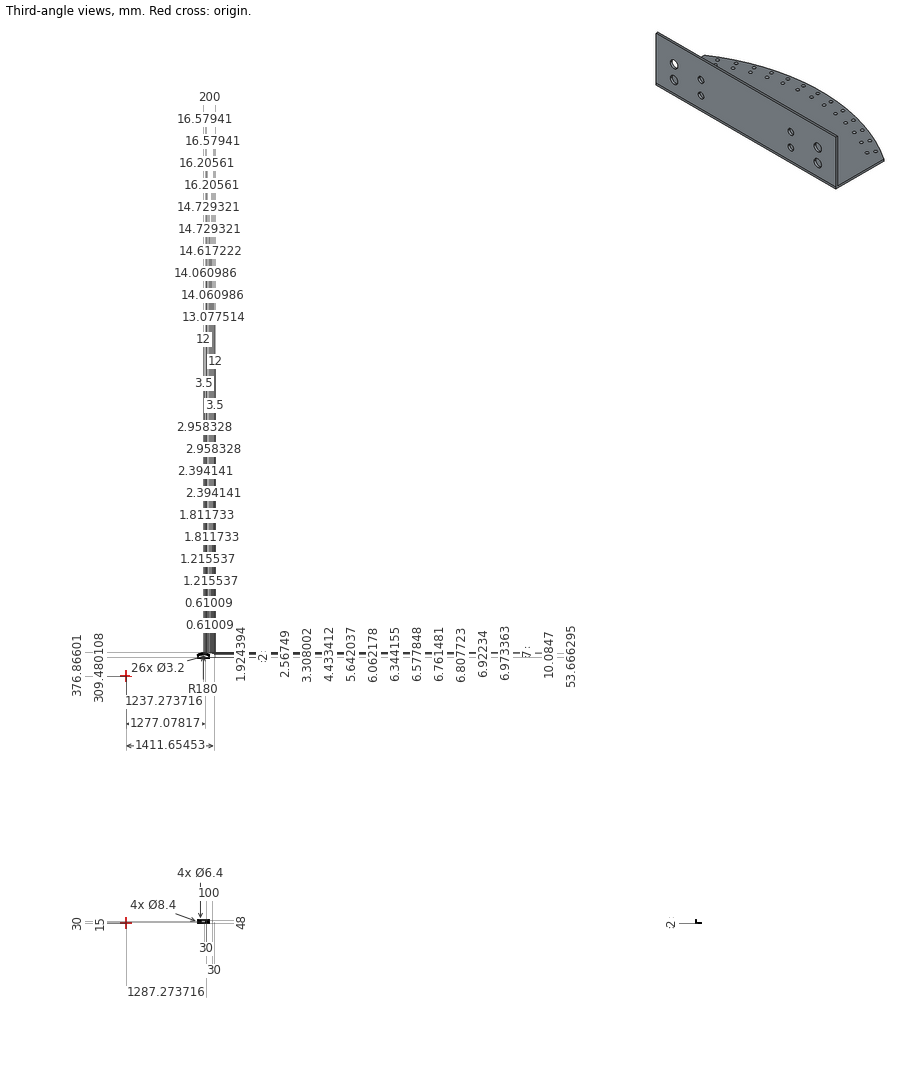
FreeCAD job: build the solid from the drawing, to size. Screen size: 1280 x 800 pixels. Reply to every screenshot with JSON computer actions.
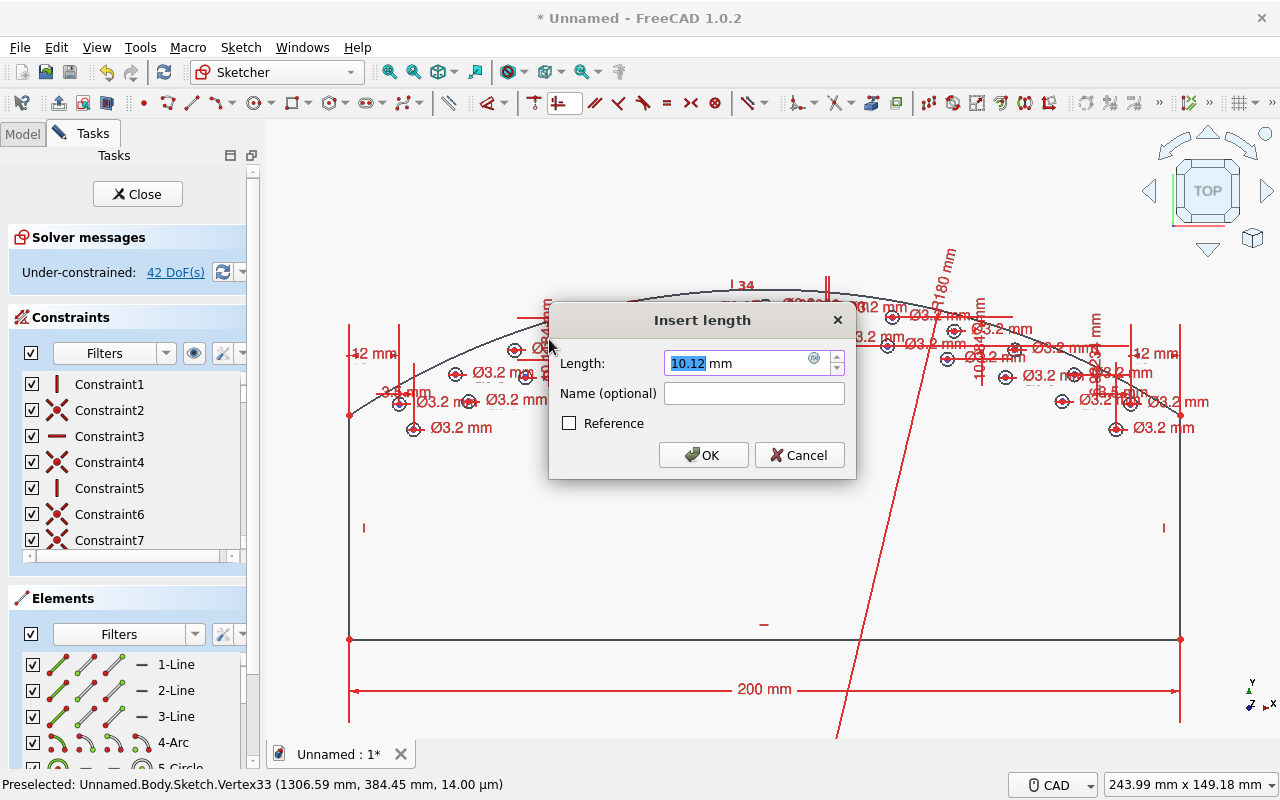
{"action": "type", "text": "10.0847"}
{"action": "key", "text": "Return"}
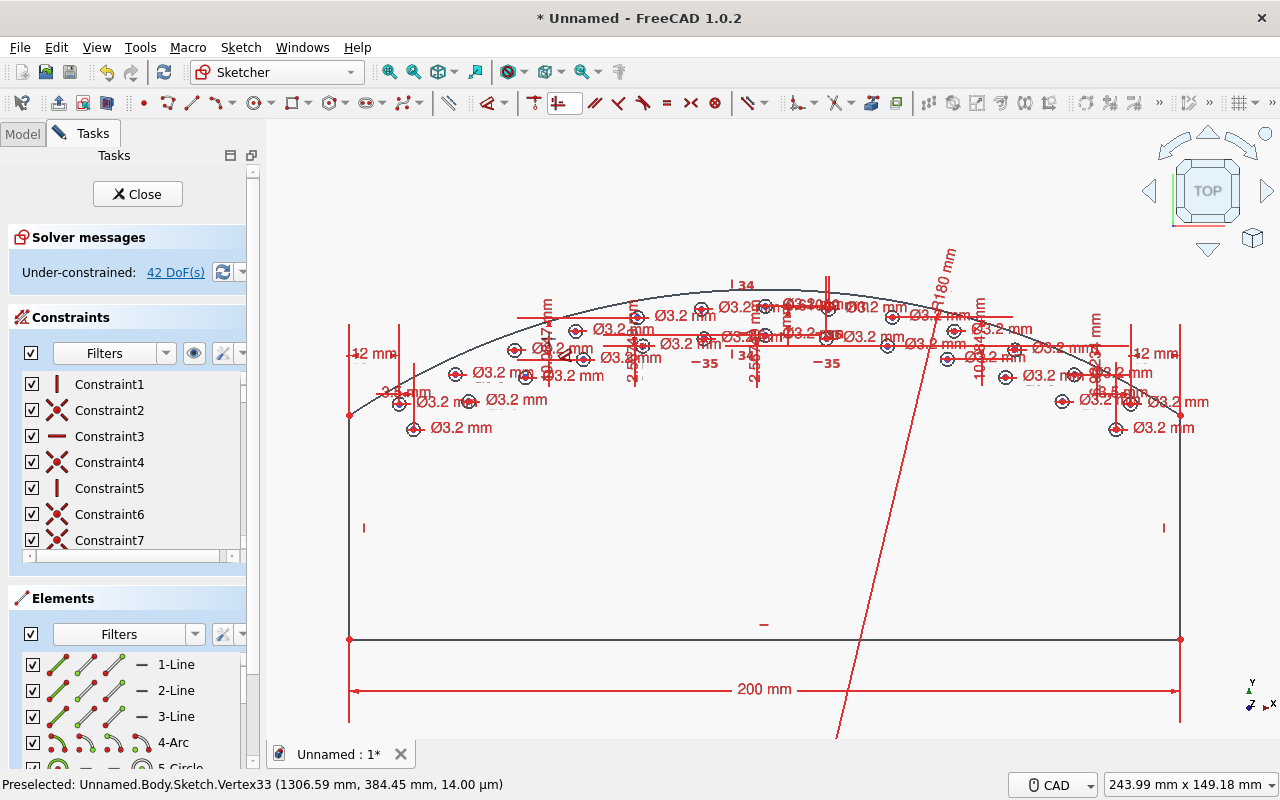
{"action": "scroll", "coordinate": [704, 339], "scroll_direction": "up", "scroll_amount": 14}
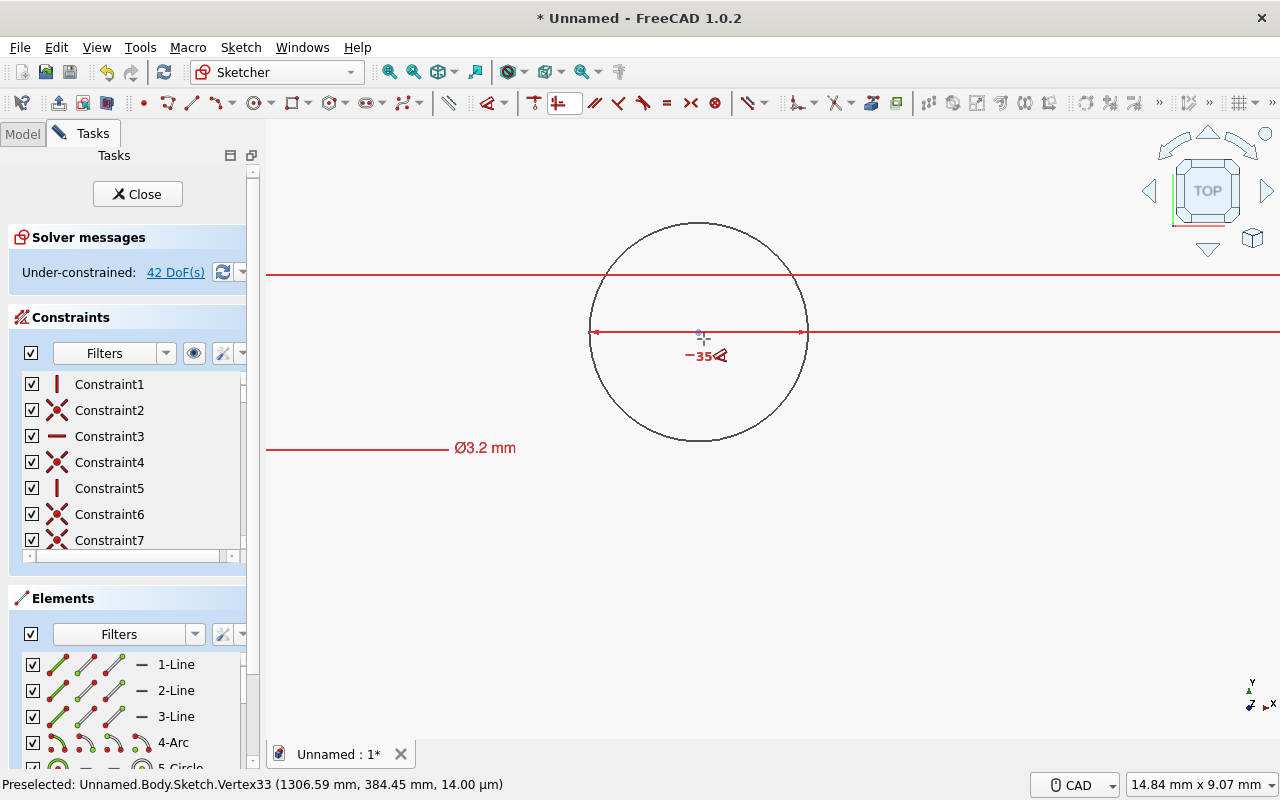
{"action": "left_click", "coordinate": [699, 332]}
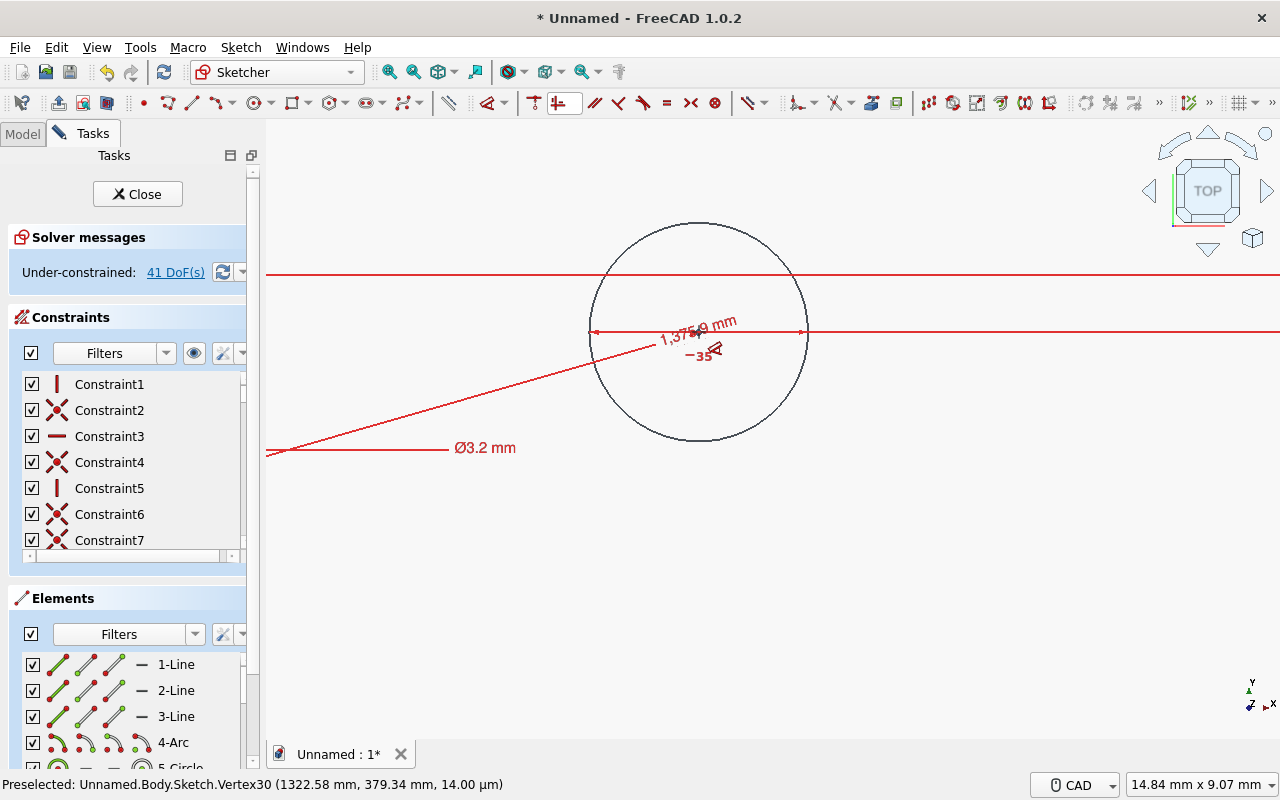
{"action": "scroll", "coordinate": [652, 327], "scroll_direction": "down", "scroll_amount": 15}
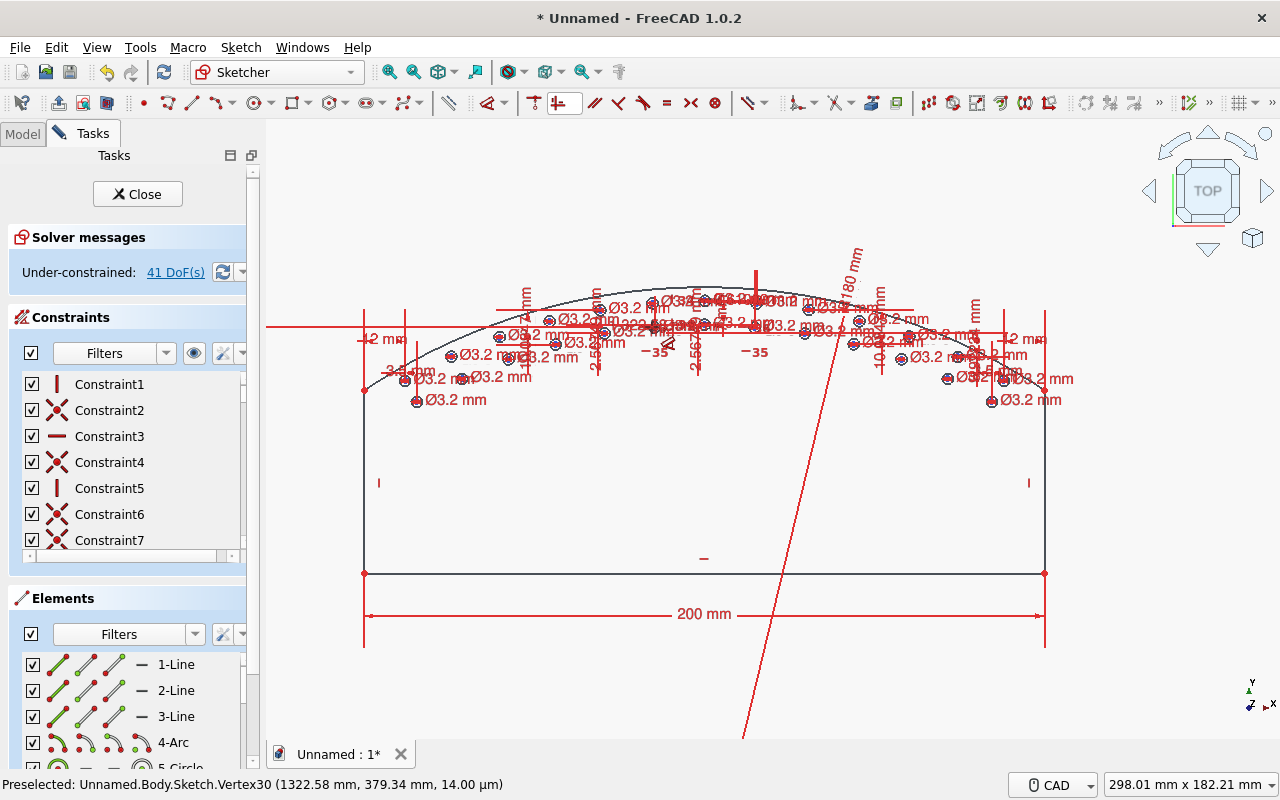
{"action": "scroll", "coordinate": [653, 303], "scroll_direction": "up", "scroll_amount": 15}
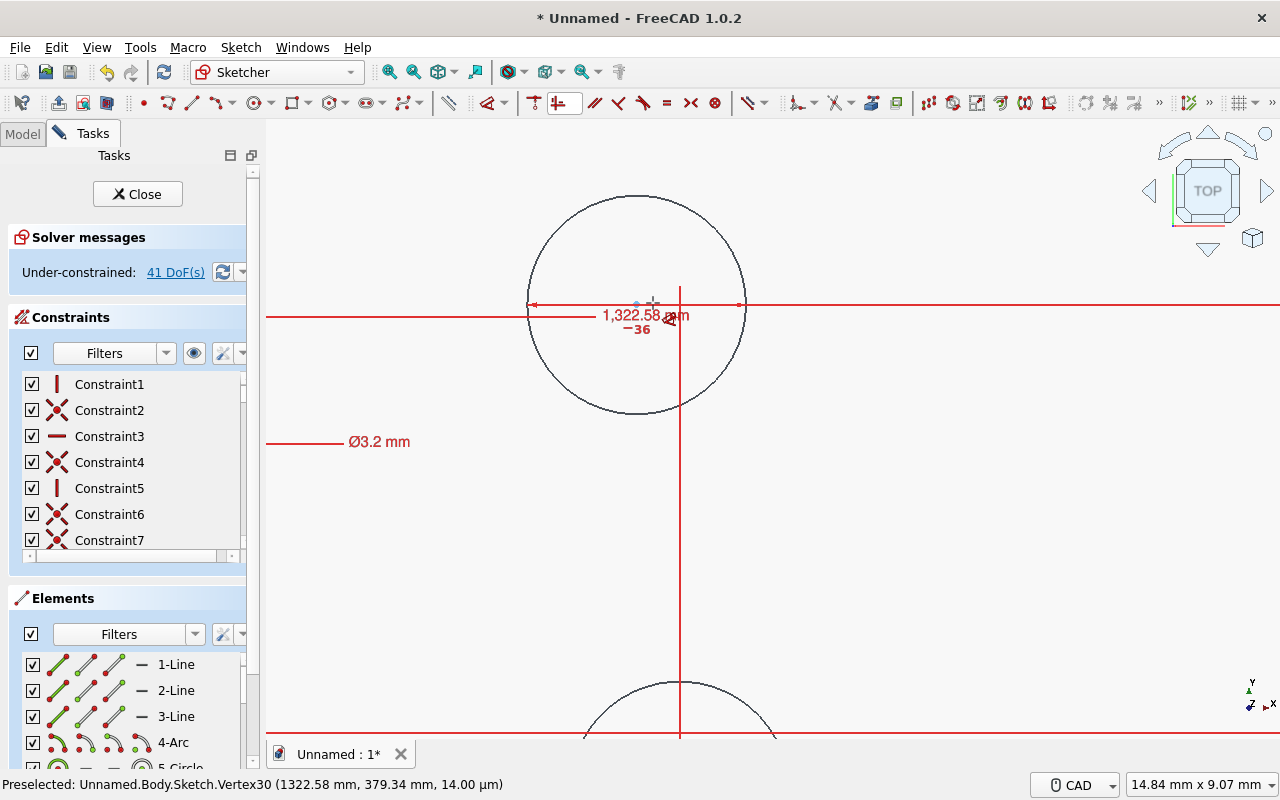
{"action": "left_click", "coordinate": [637, 305]}
{"action": "left_click", "coordinate": [658, 271]}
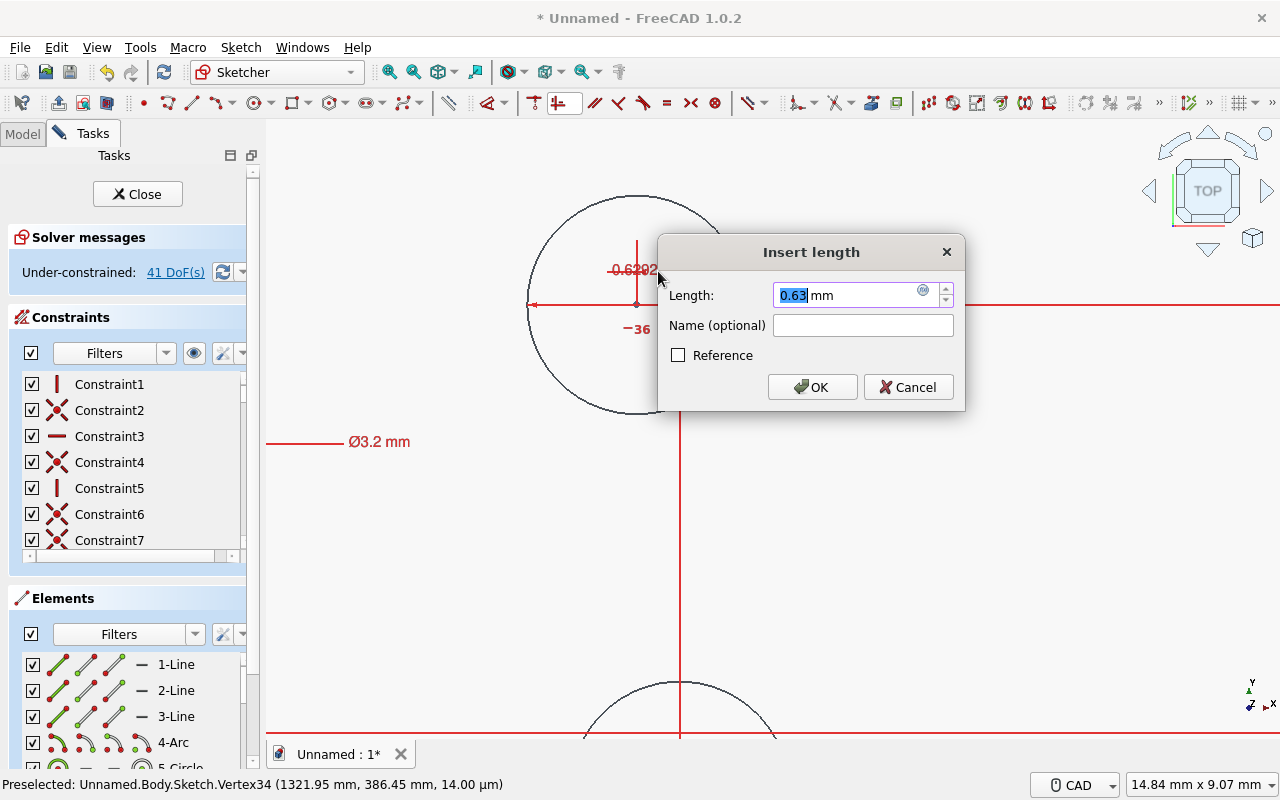
{"action": "type", "text": "0.61009"}
{"action": "key", "text": "Return"}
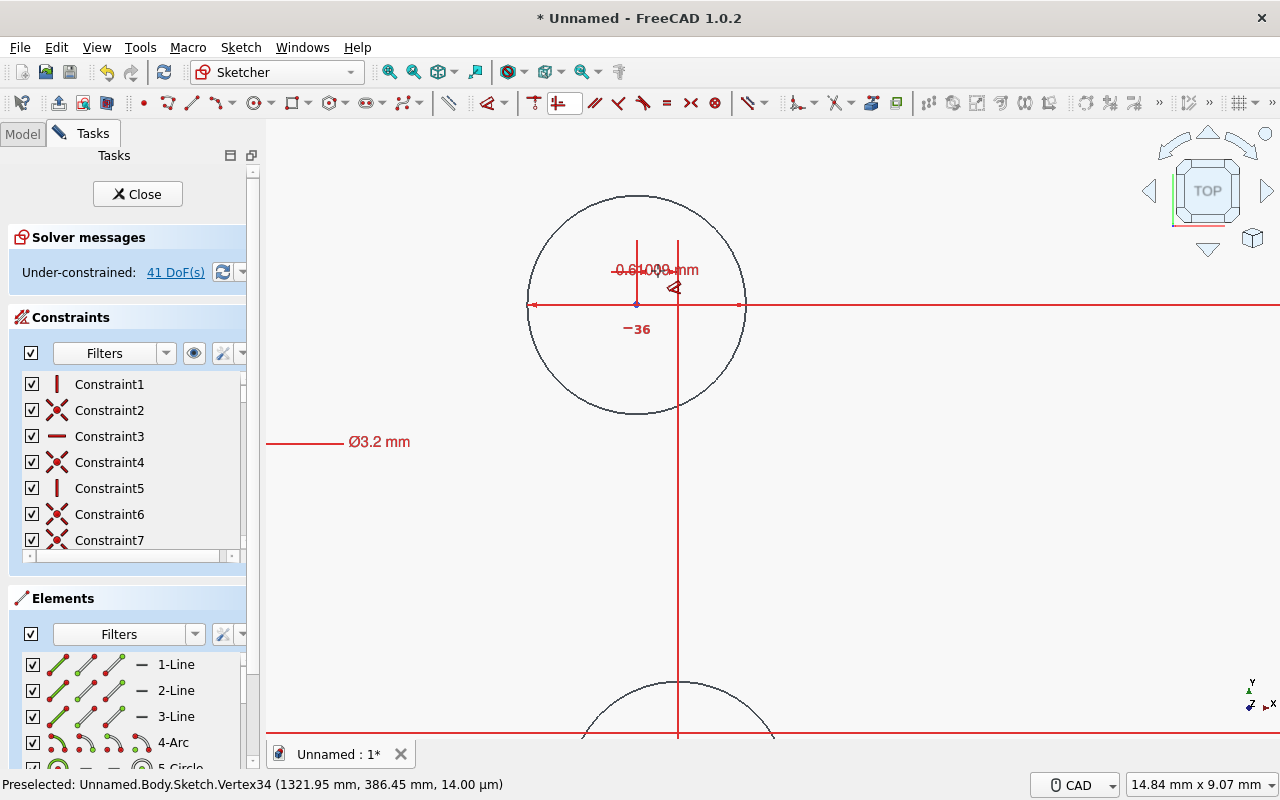
{"action": "scroll", "coordinate": [653, 303], "scroll_direction": "down", "scroll_amount": 15}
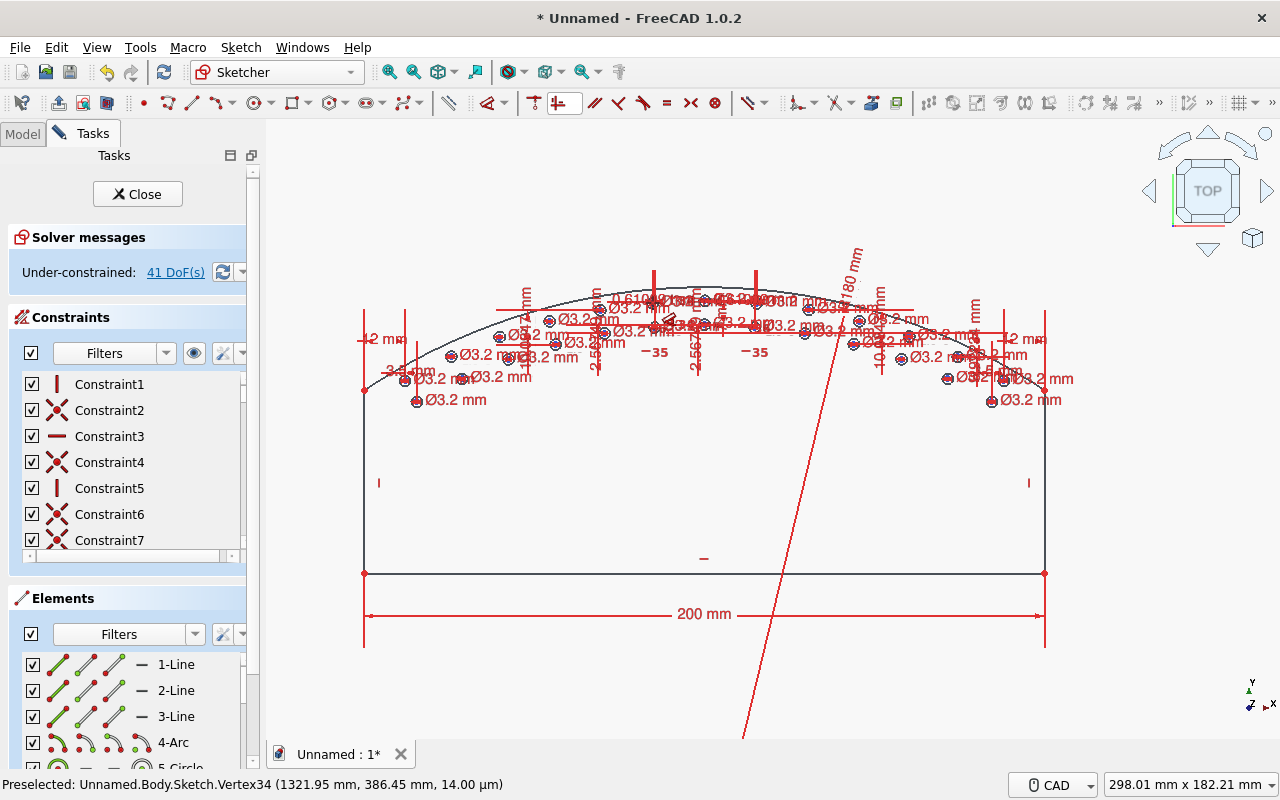
{"action": "left_click", "coordinate": [364, 445]}
{"action": "left_click", "coordinate": [330, 482]}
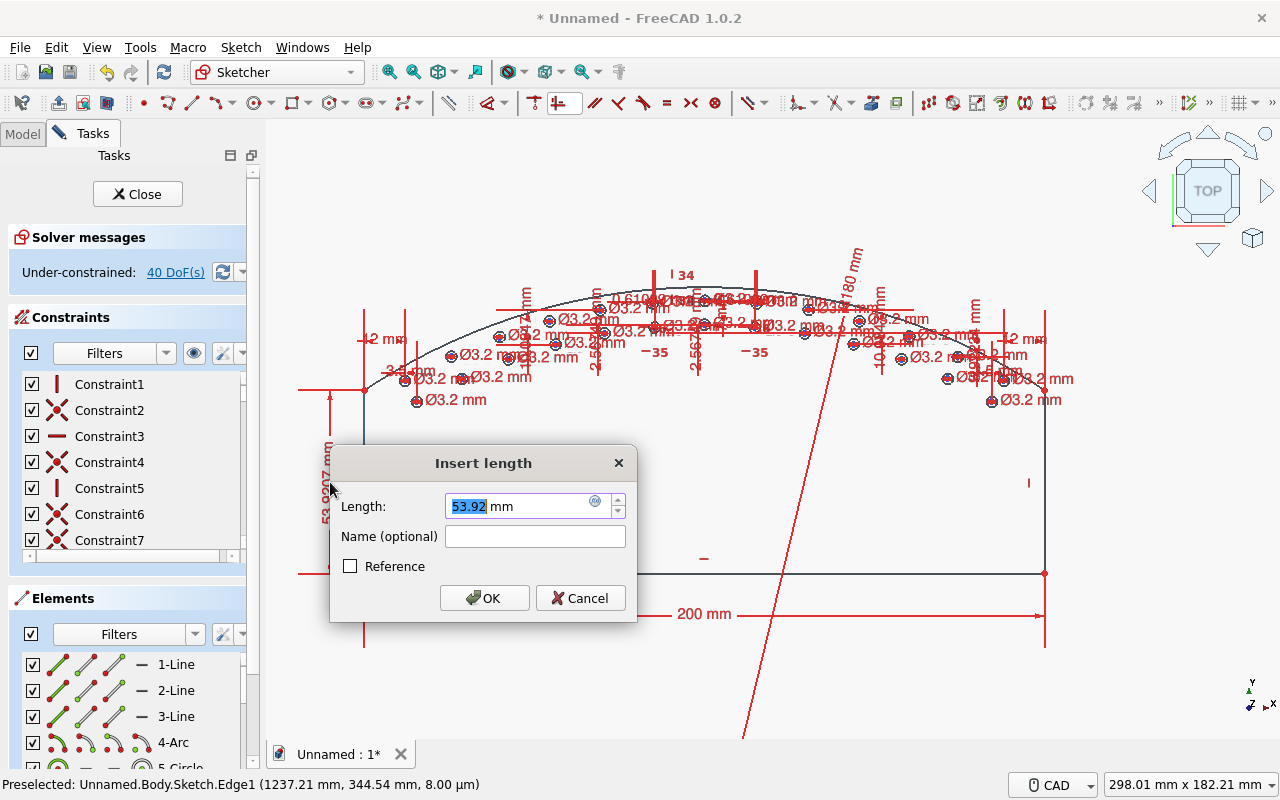
{"action": "type", "text": "53.666295"}
{"action": "key", "text": "Return"}